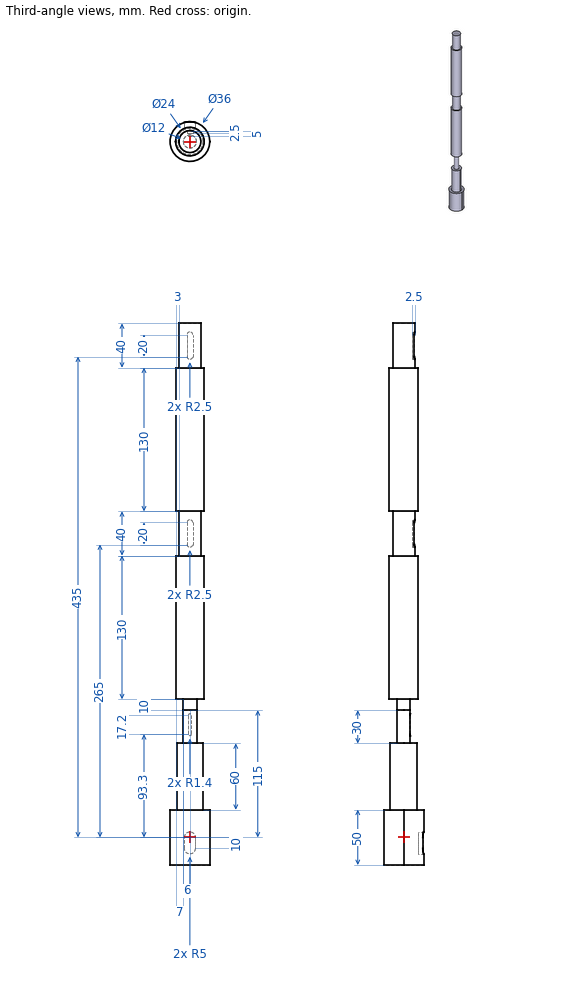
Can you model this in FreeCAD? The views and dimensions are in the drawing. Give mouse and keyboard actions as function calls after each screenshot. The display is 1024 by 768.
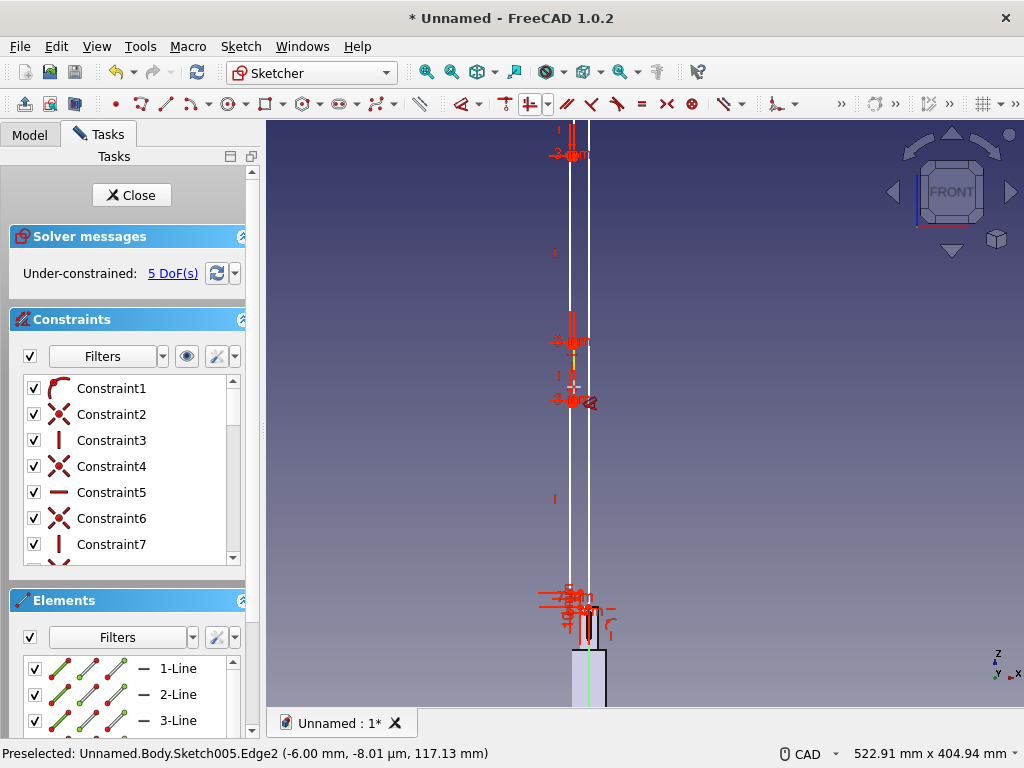
click(574, 387)
click(540, 375)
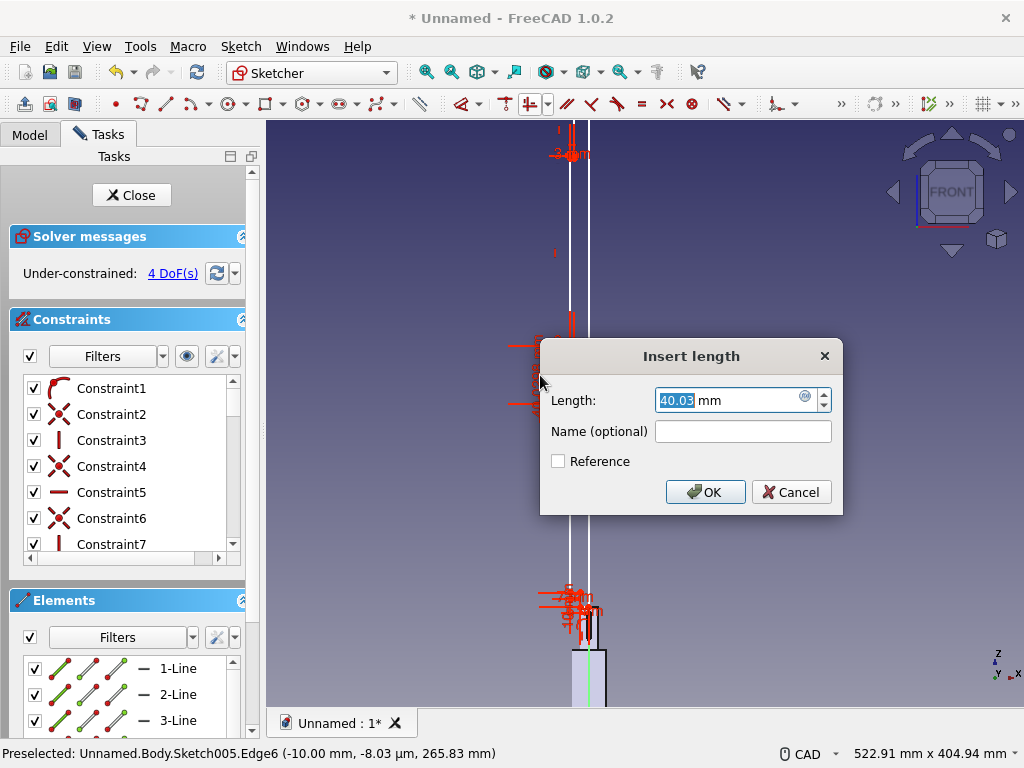
text(40)
key(Return)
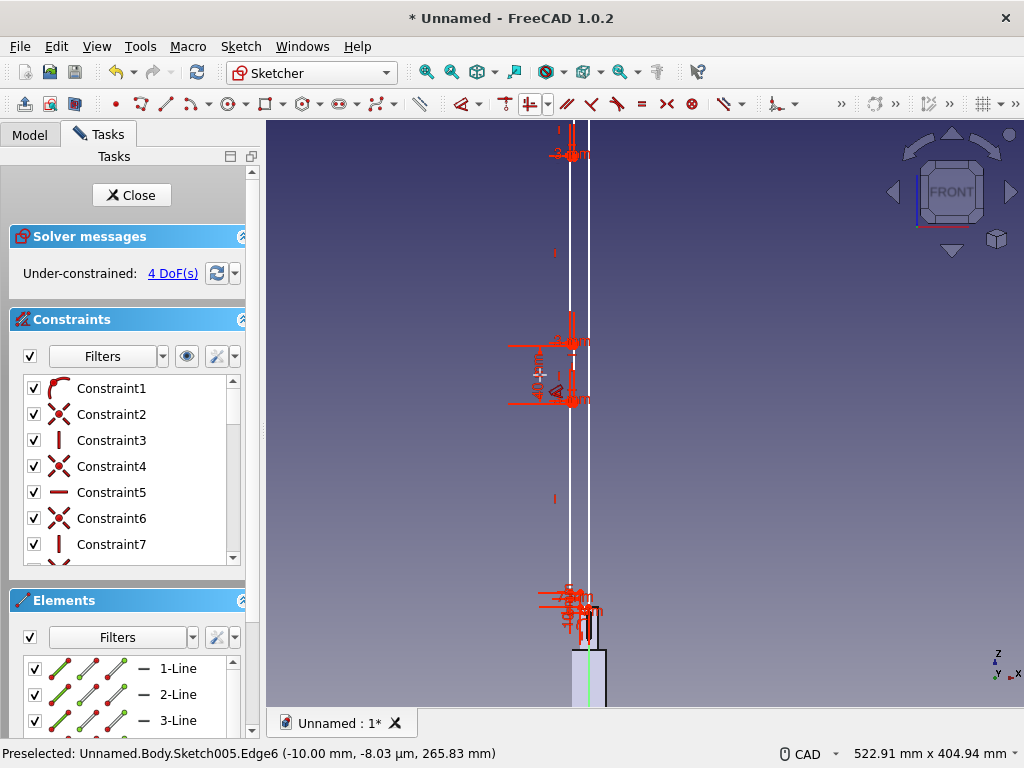
scroll(573, 386, down, 3)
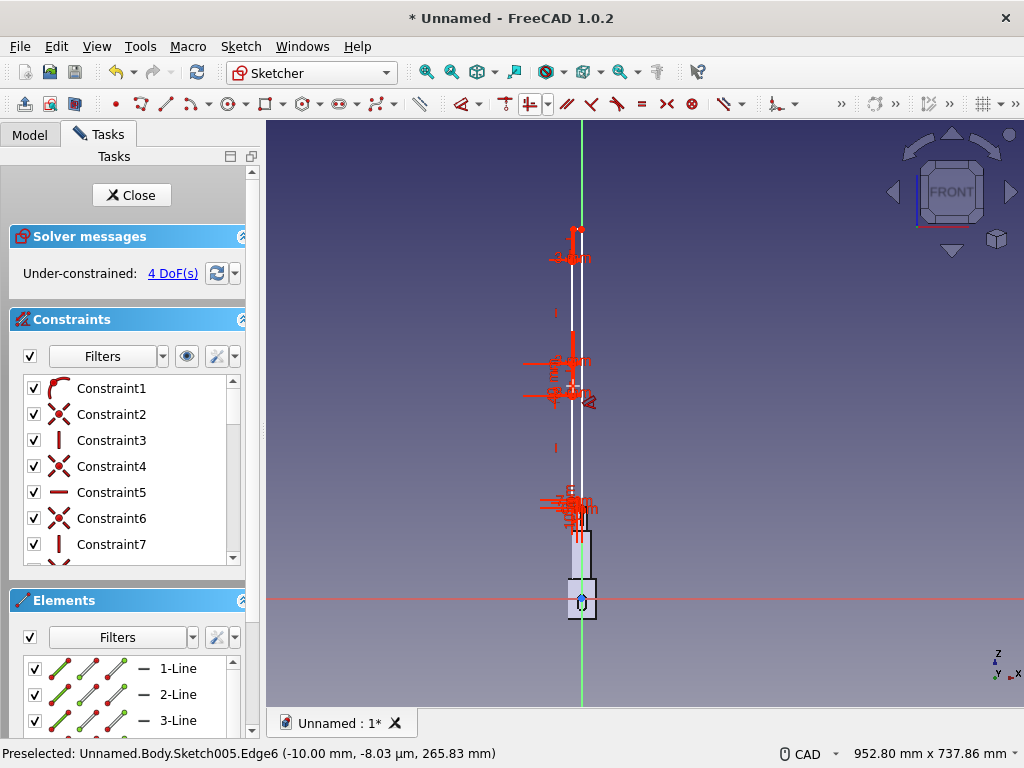
scroll(574, 252, up, 3)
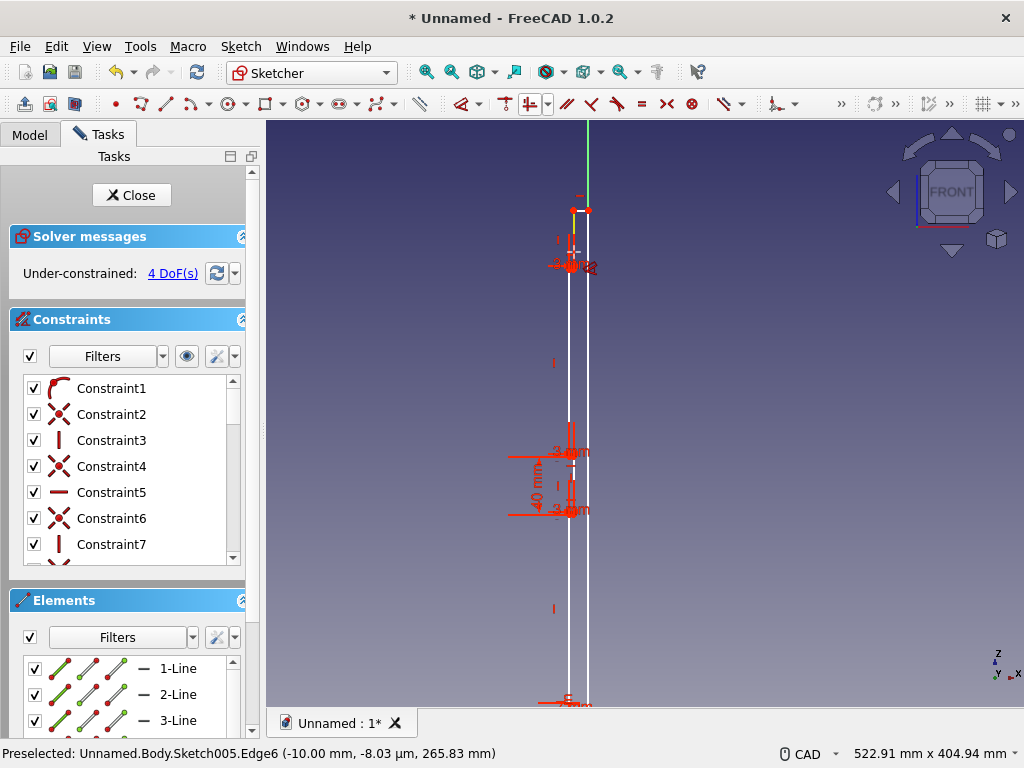
click(574, 252)
click(540, 240)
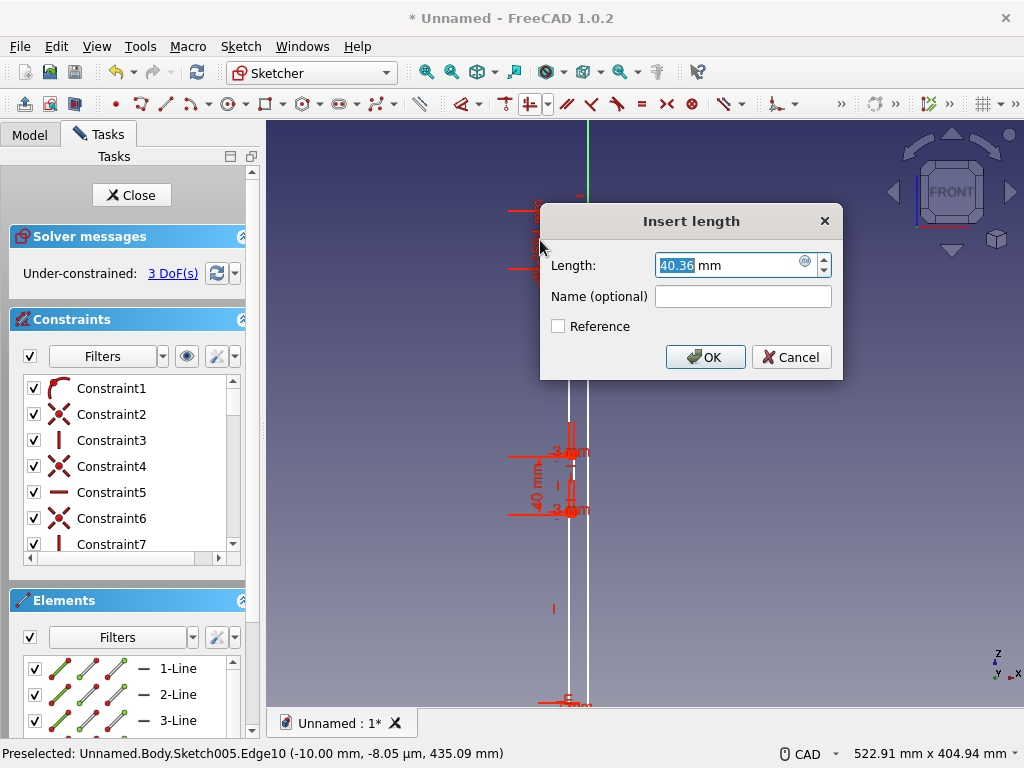
text(40)
key(Return)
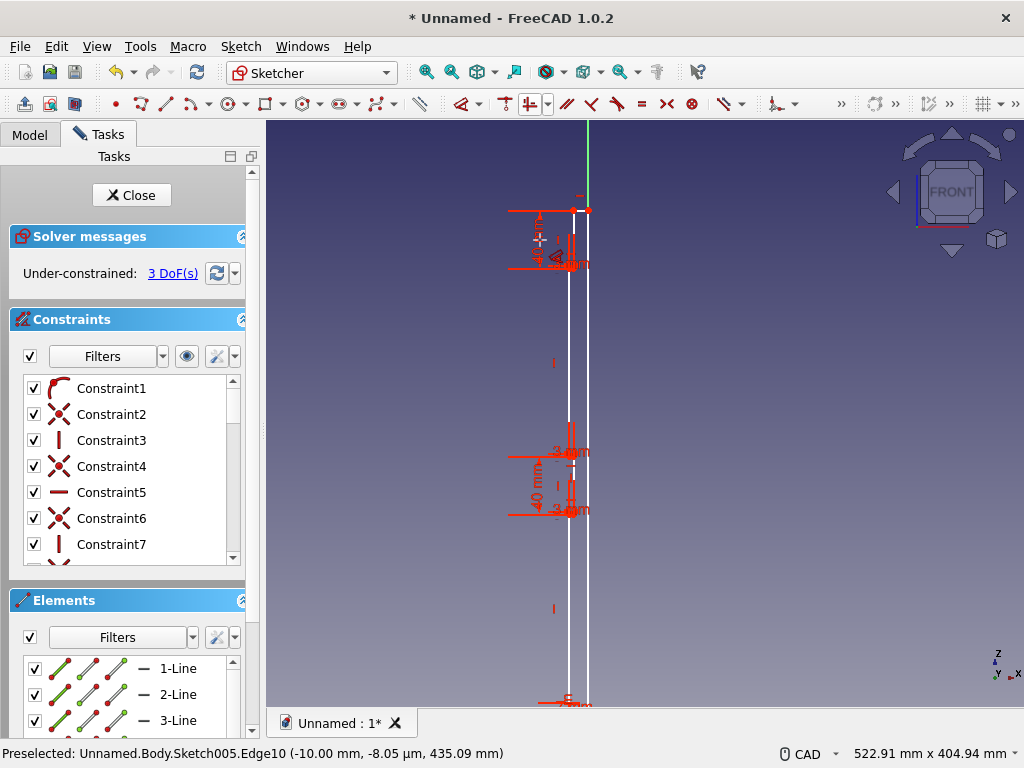
click(569, 647)
click(535, 597)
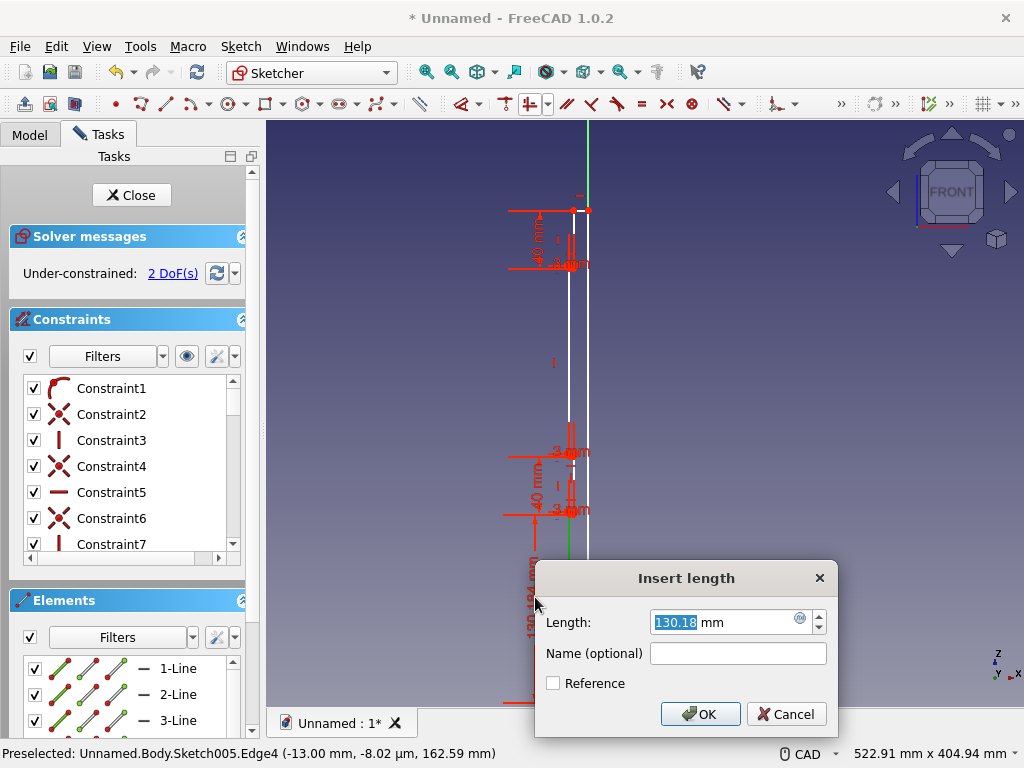
text(130)
key(Return)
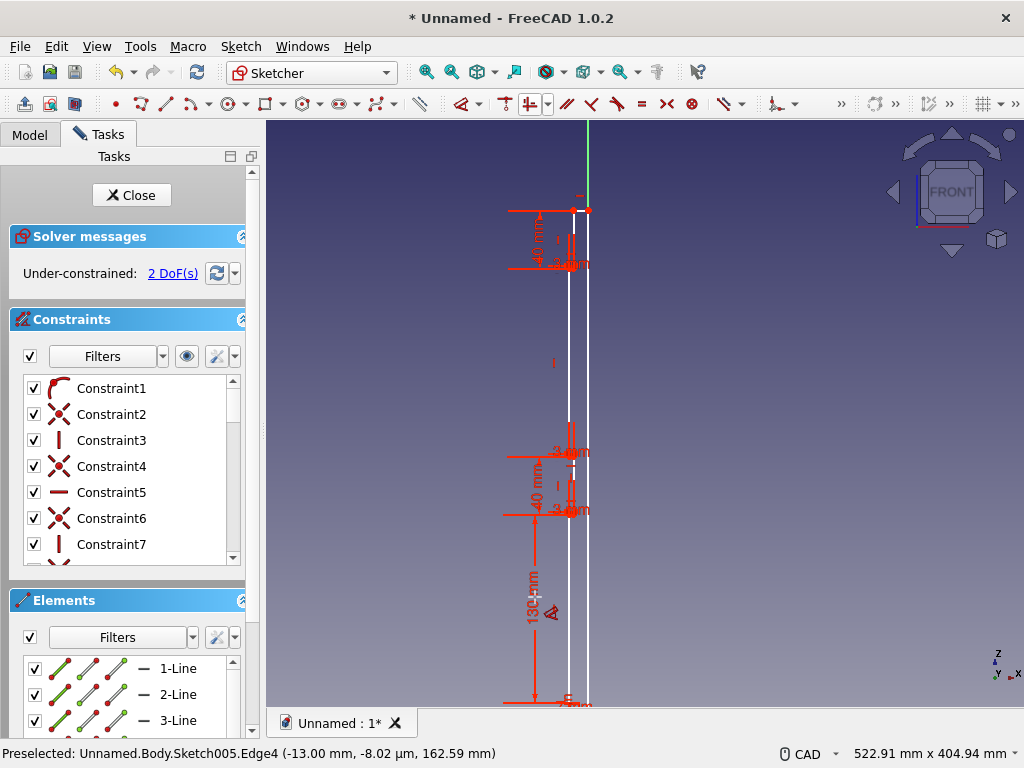
click(569, 400)
click(535, 363)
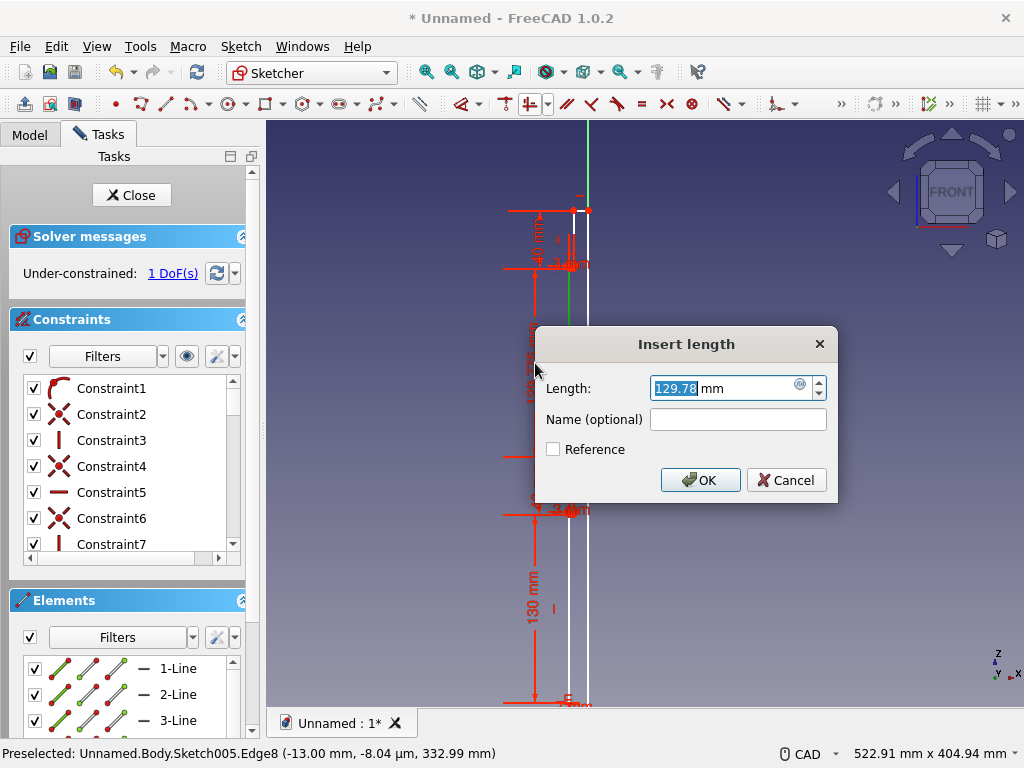
text(130)
key(Return)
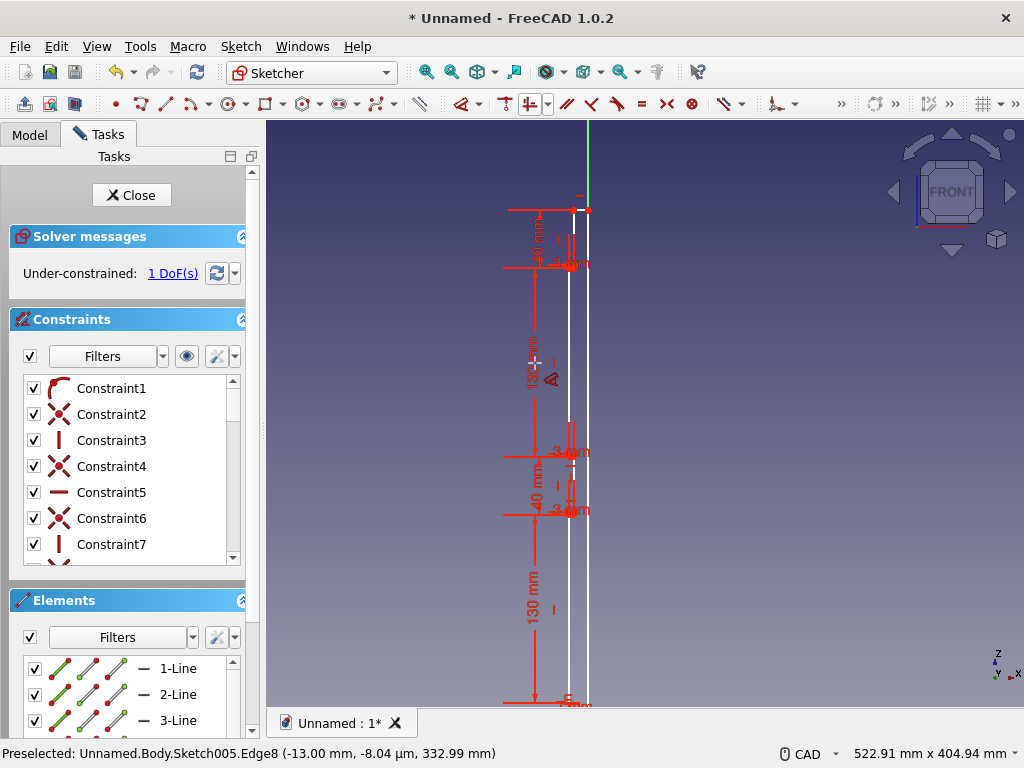
scroll(574, 252, down, 3)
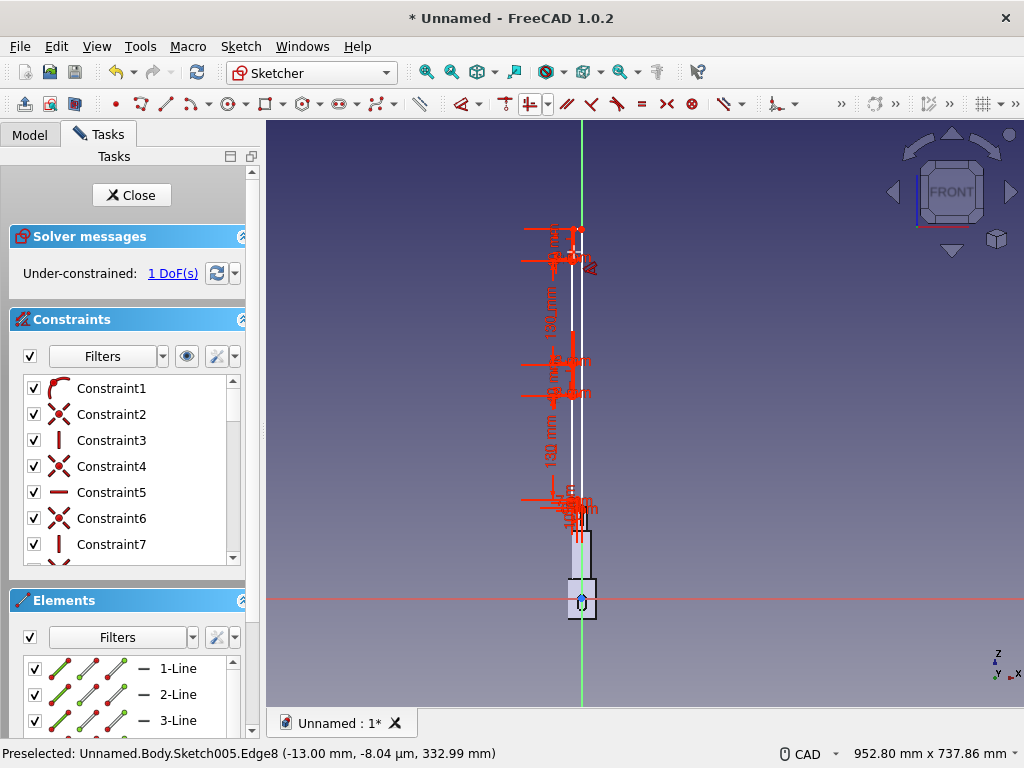
scroll(582, 508, up, 5)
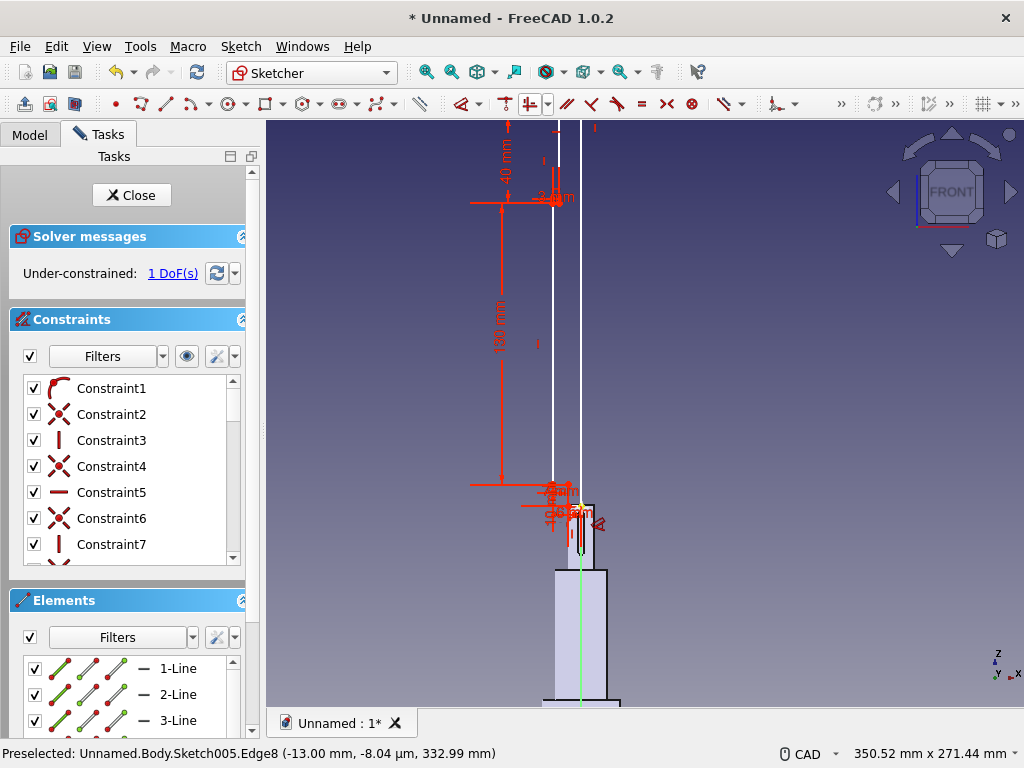
click(581, 506)
click(615, 593)